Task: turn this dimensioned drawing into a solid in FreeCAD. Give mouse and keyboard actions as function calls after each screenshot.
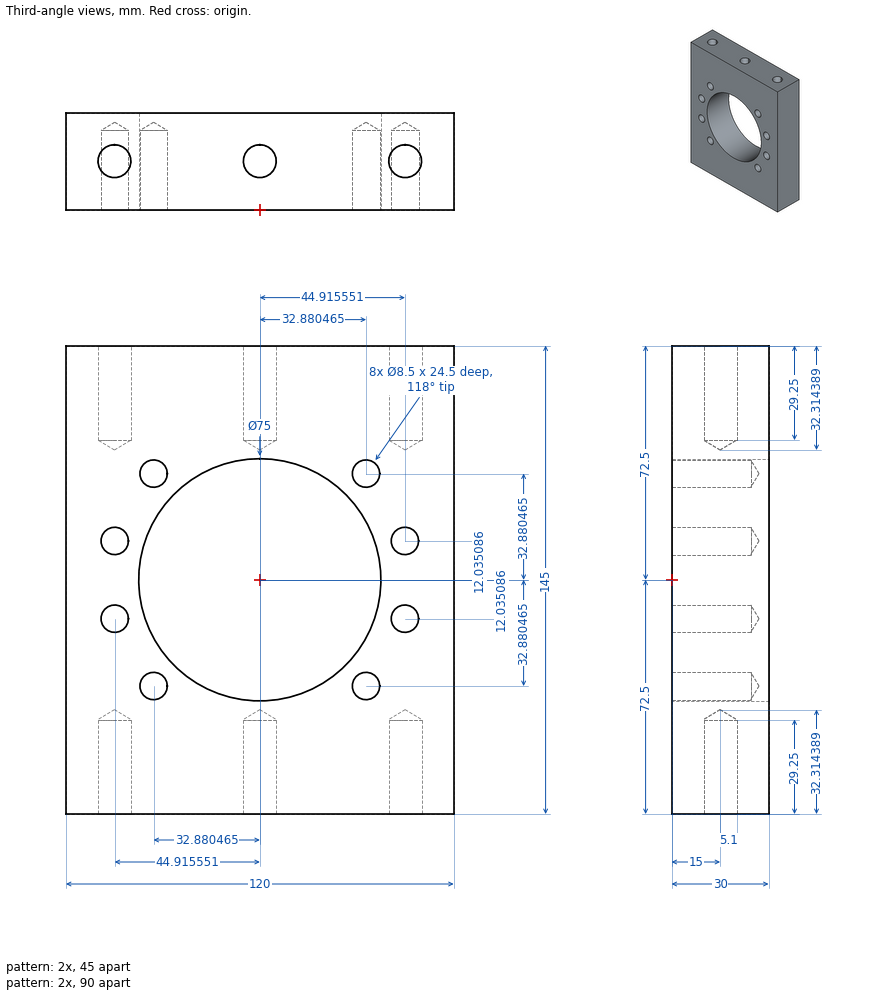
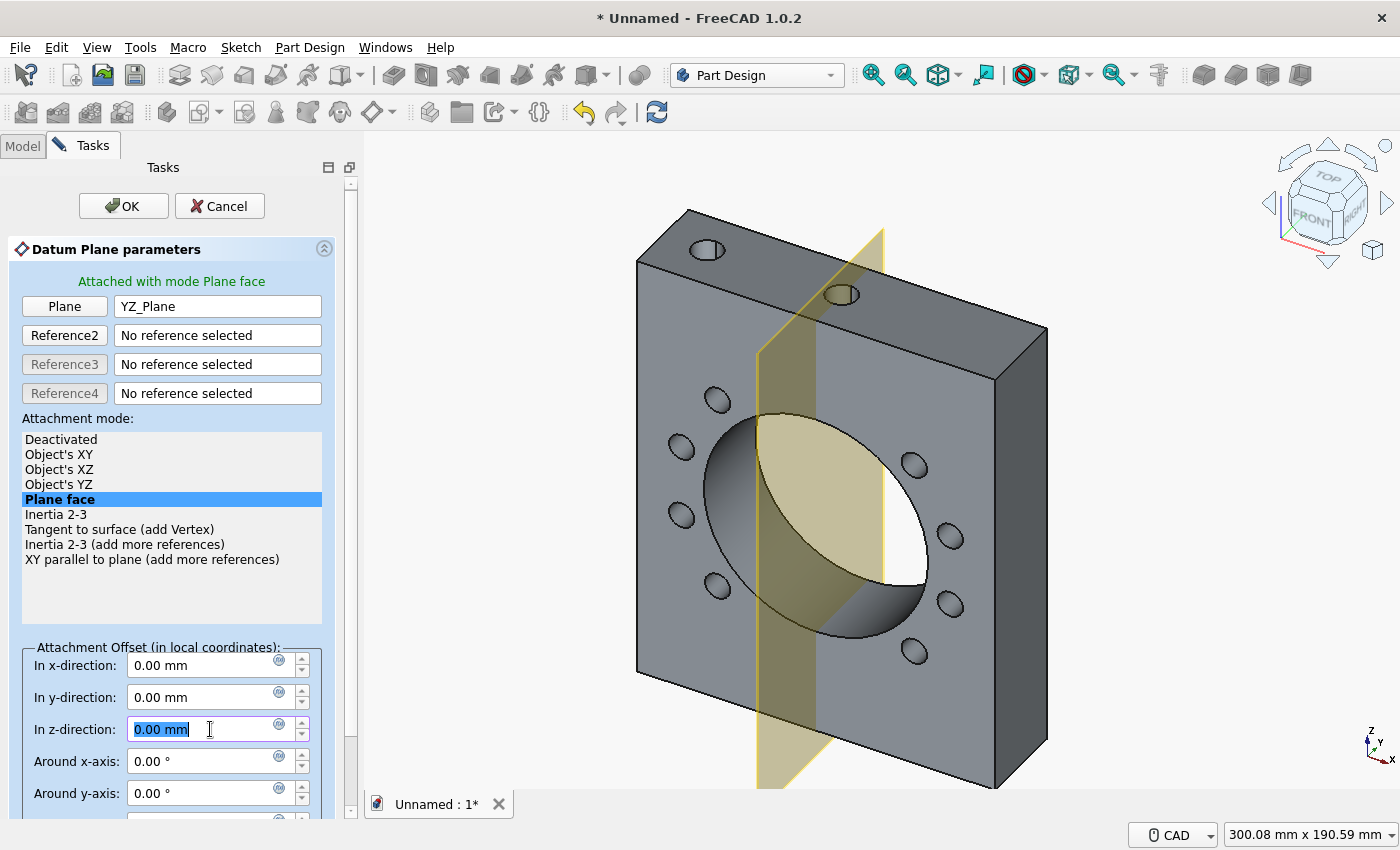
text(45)
key(Tab)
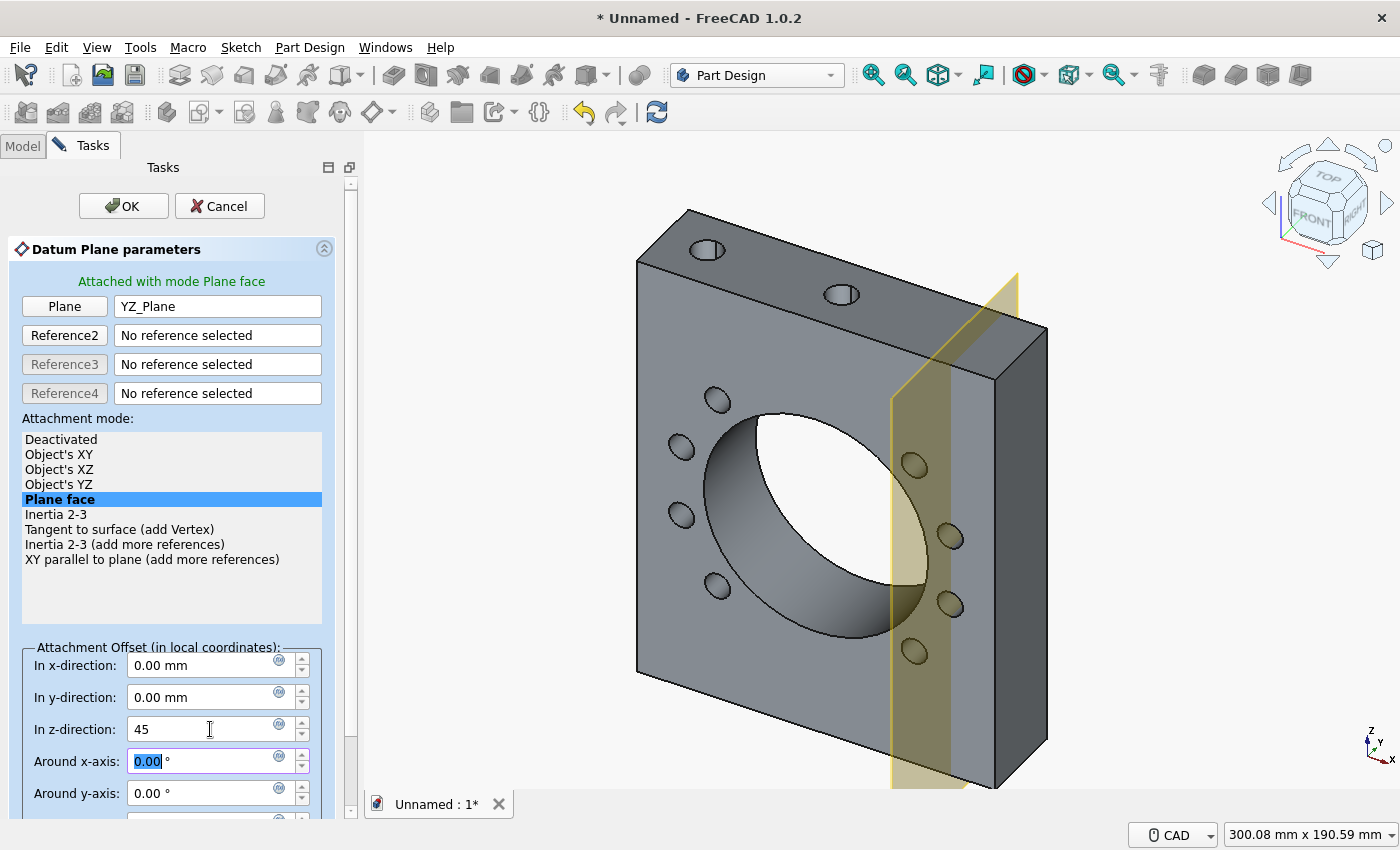
click(124, 206)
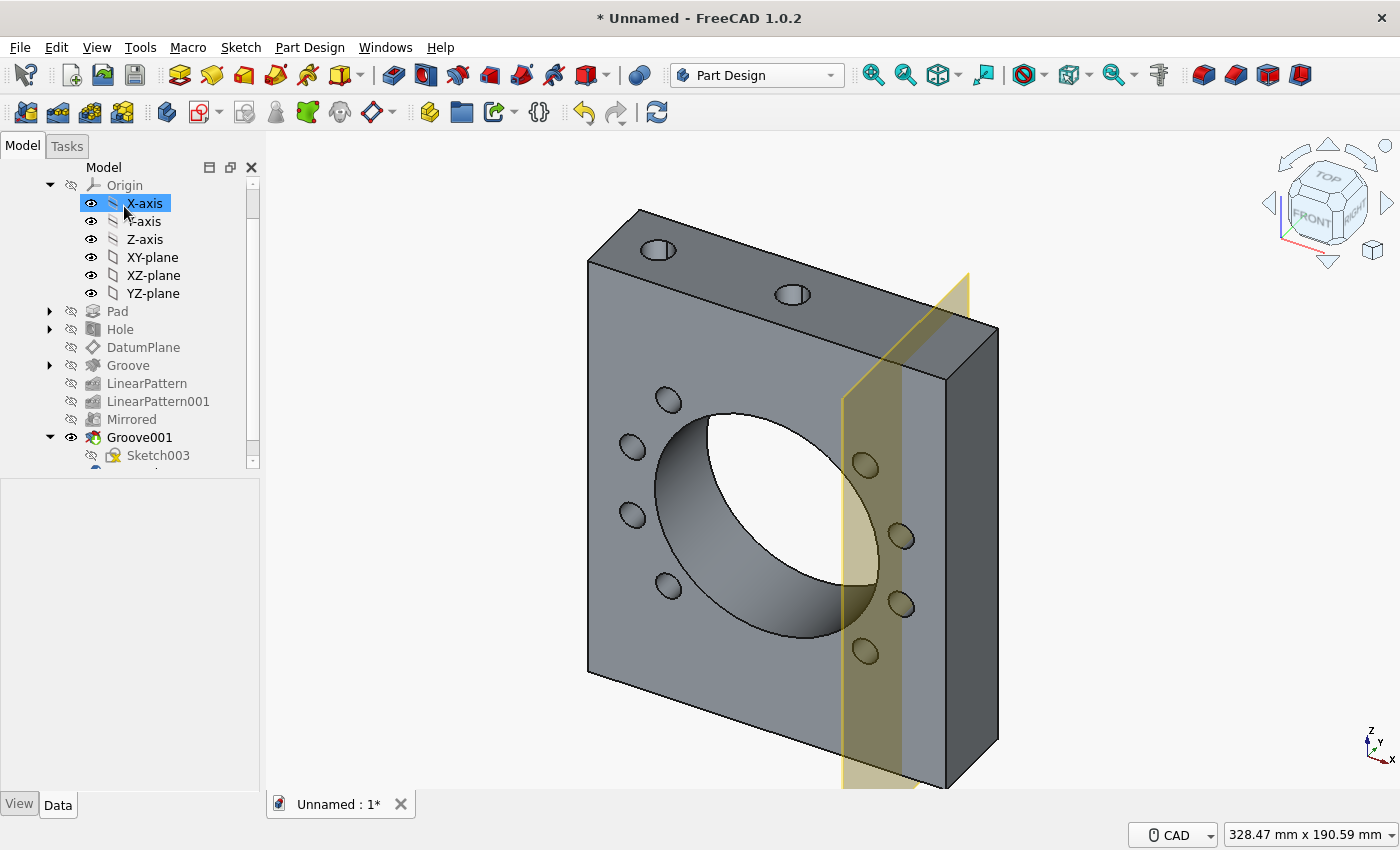
scroll(140, 325, down, 3)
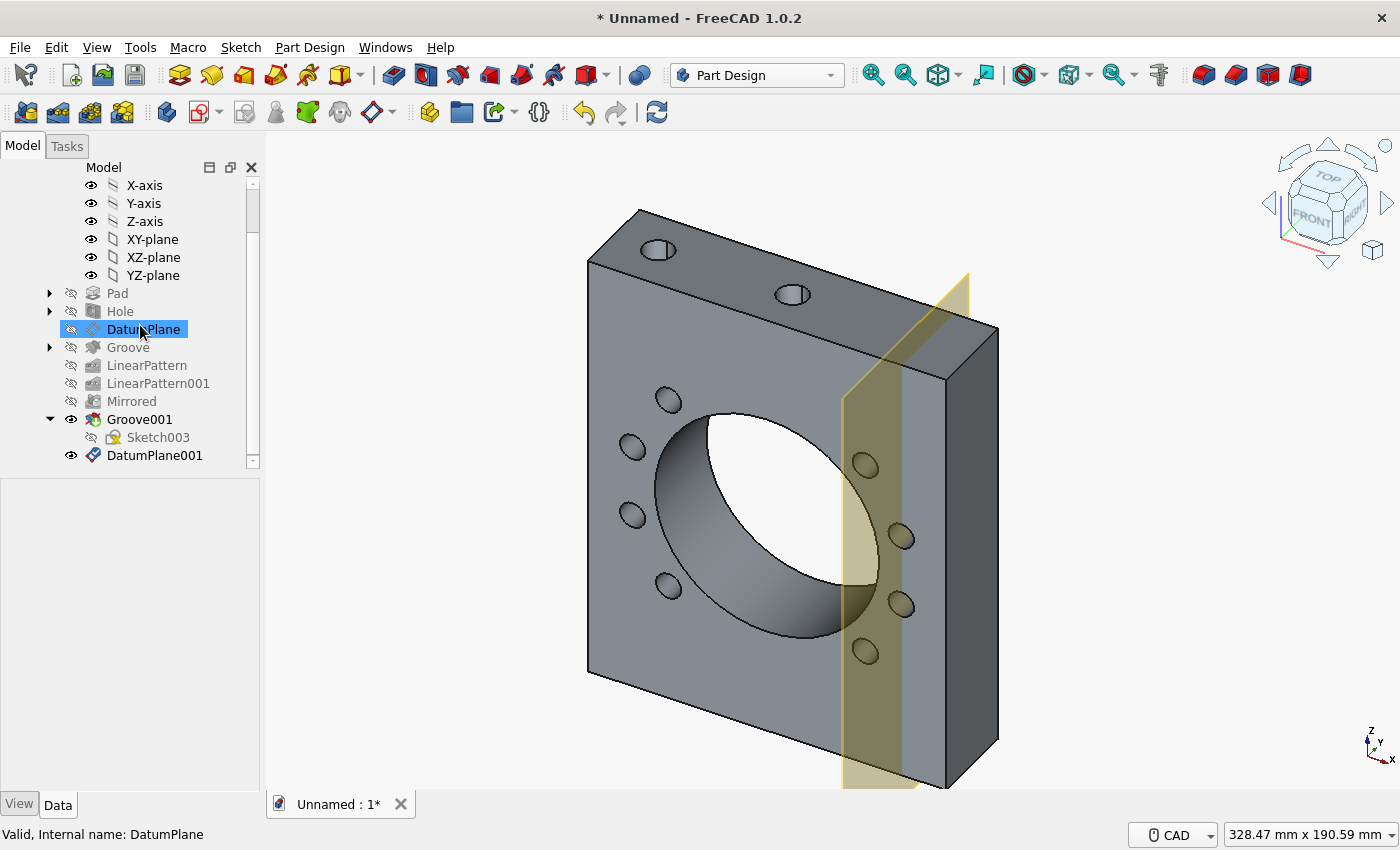
click(116, 455)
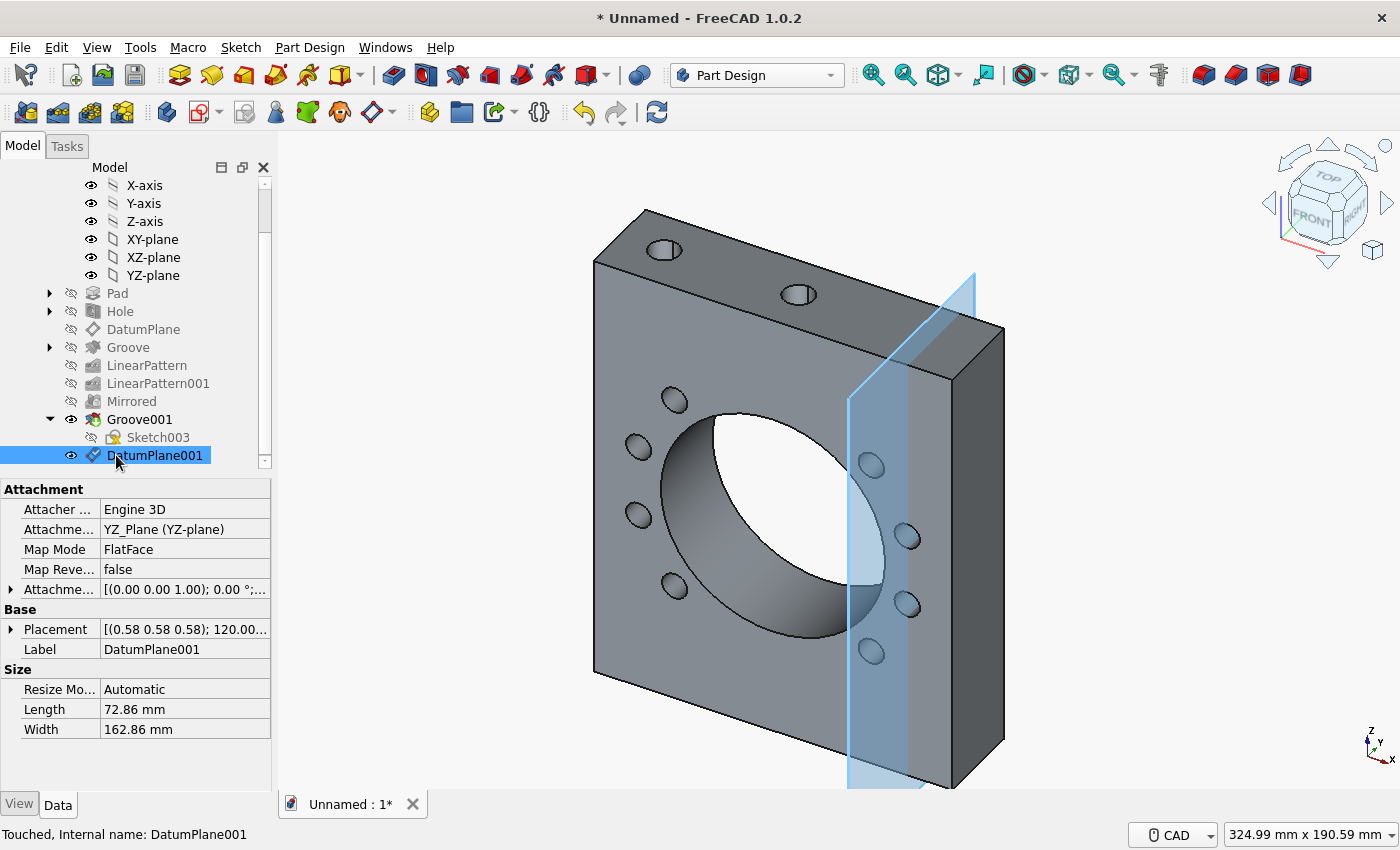
click(200, 112)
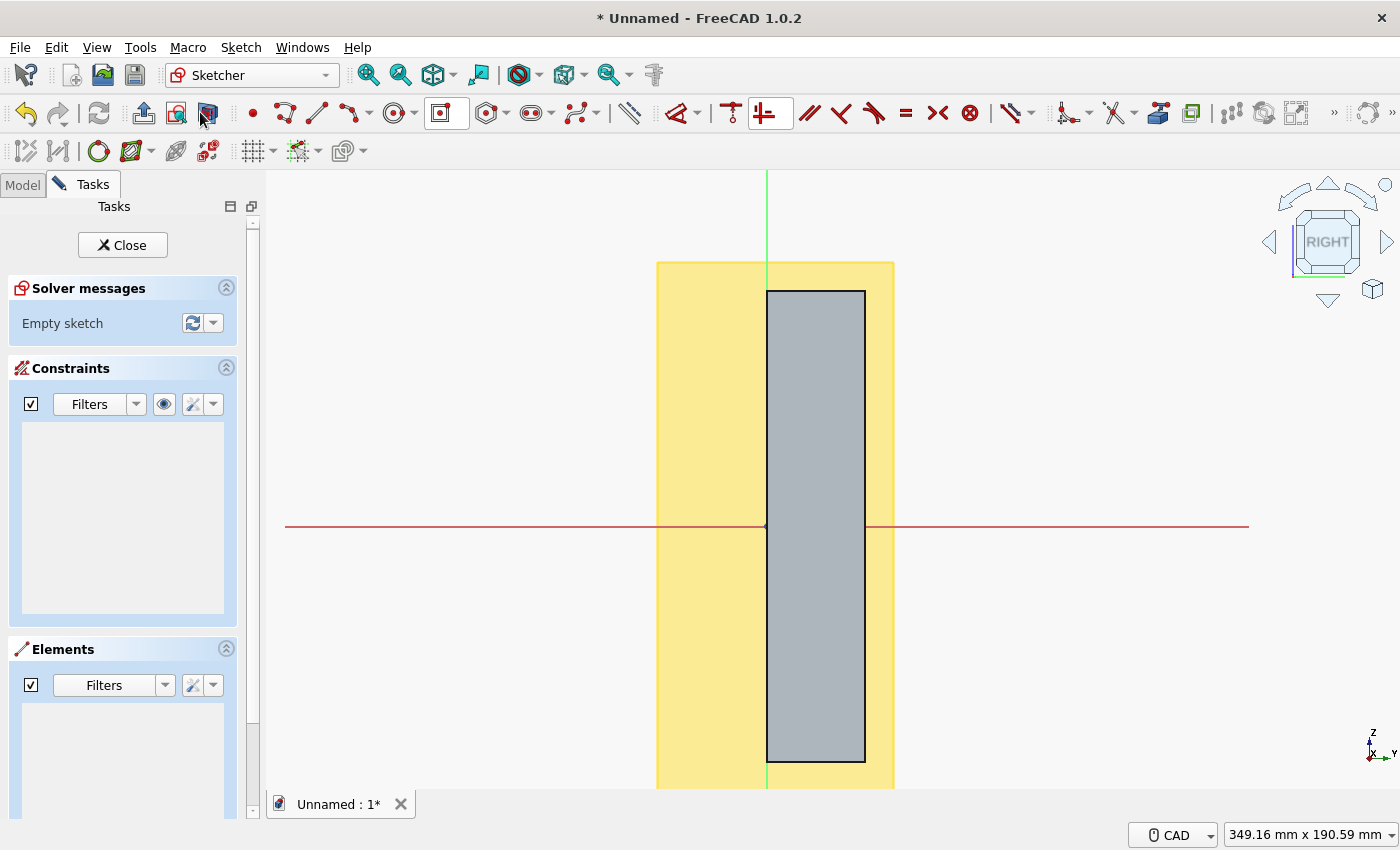
click(208, 114)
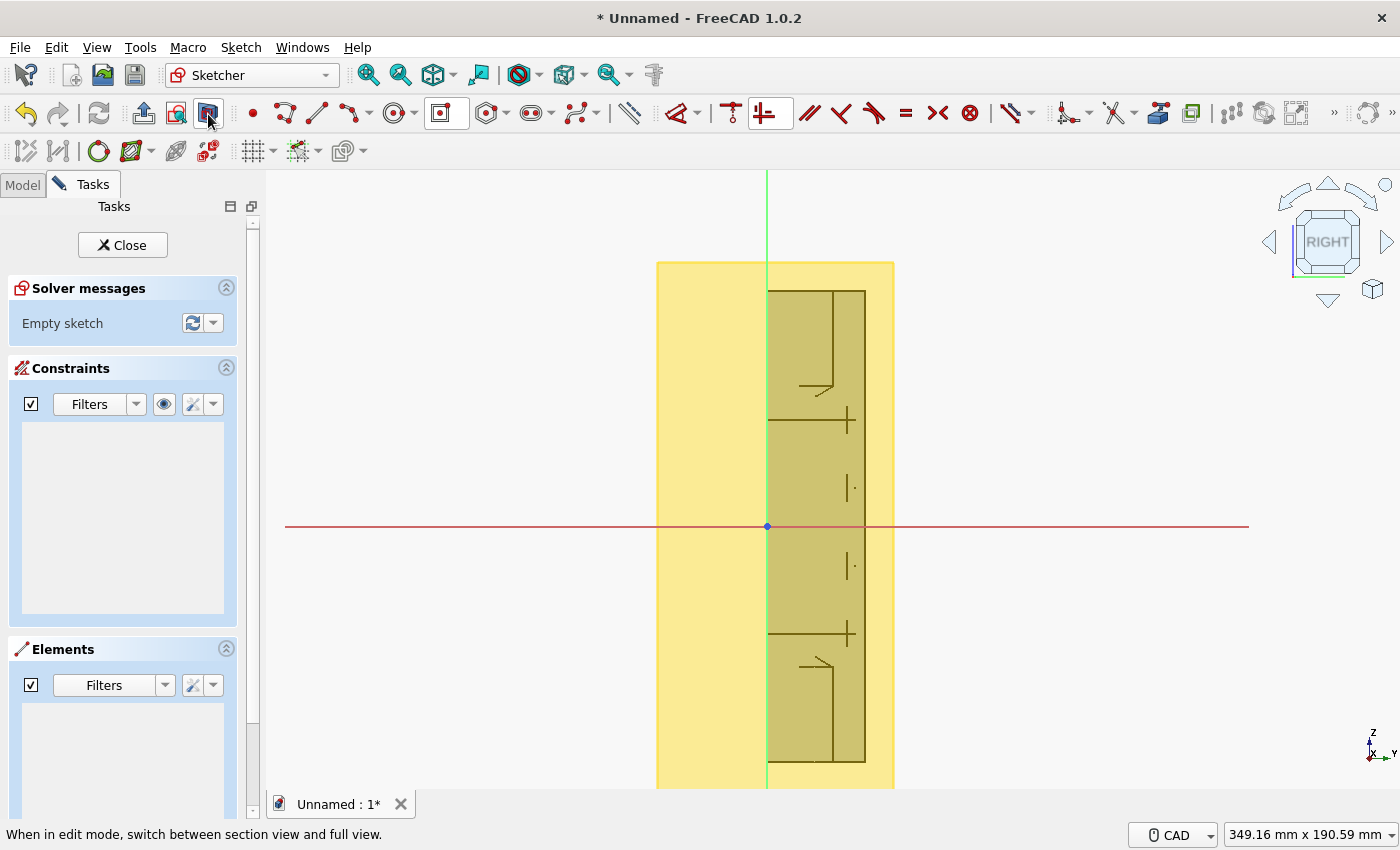
scroll(872, 203, up, 2)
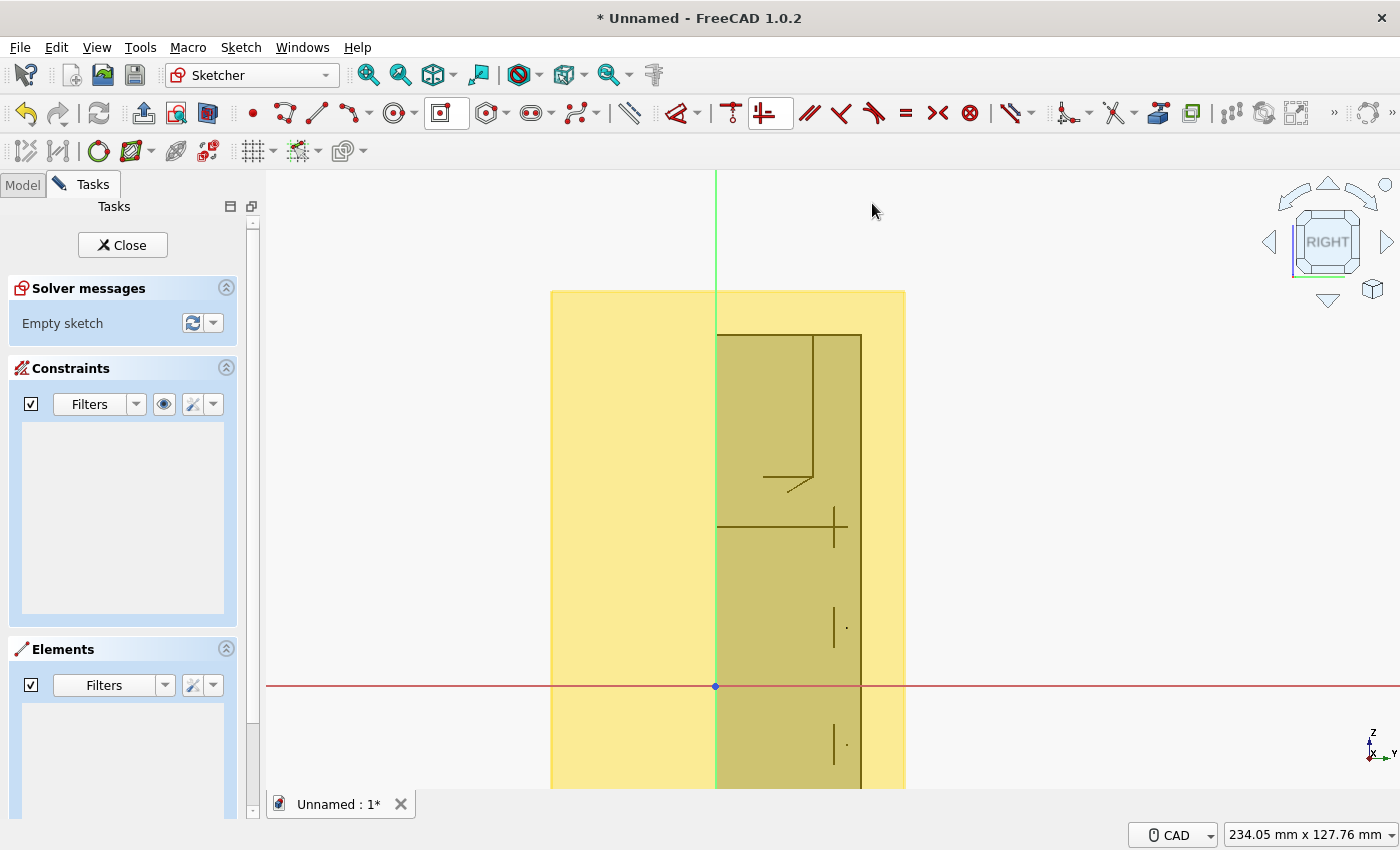
click(286, 114)